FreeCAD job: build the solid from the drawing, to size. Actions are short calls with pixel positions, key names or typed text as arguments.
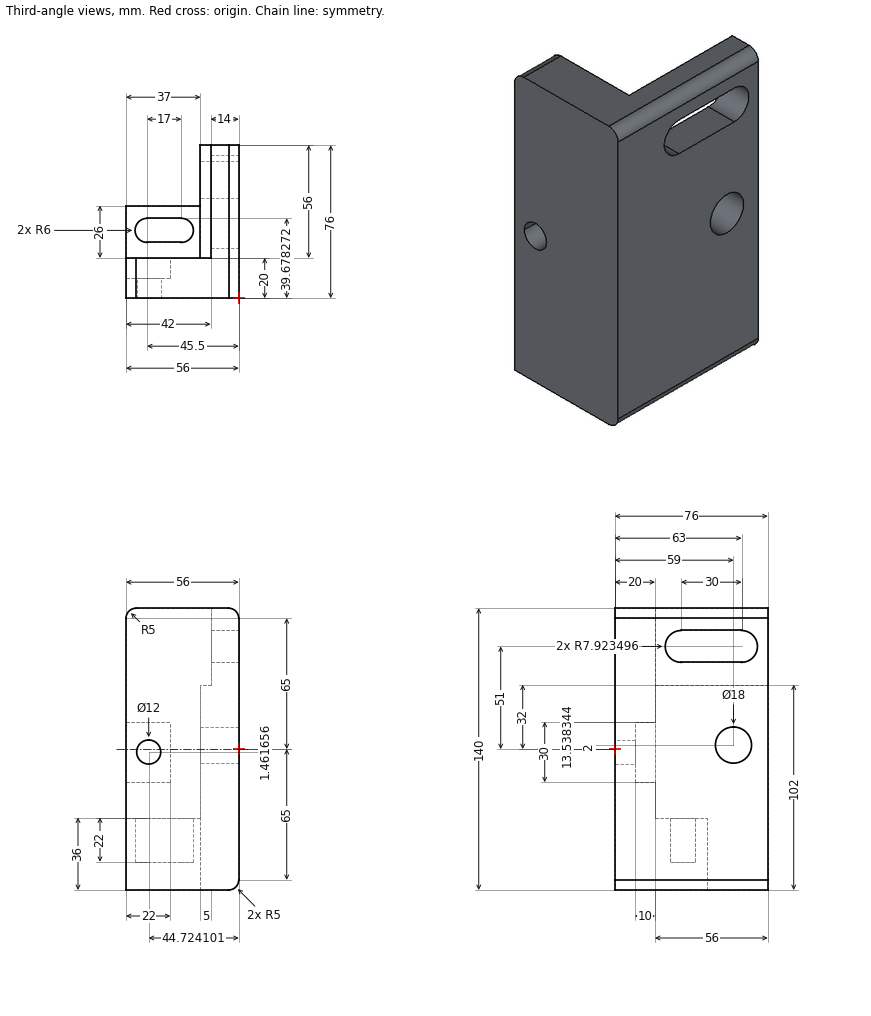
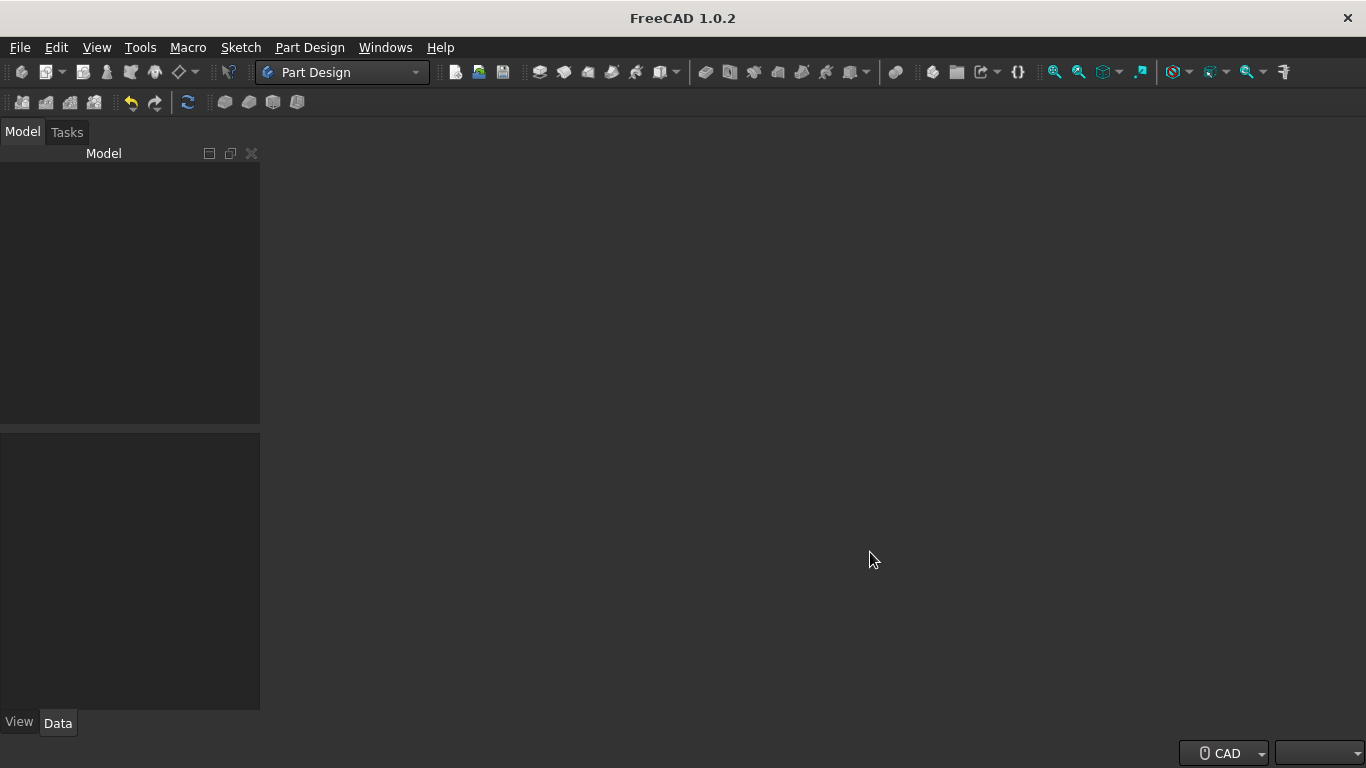
key(ctrl+n)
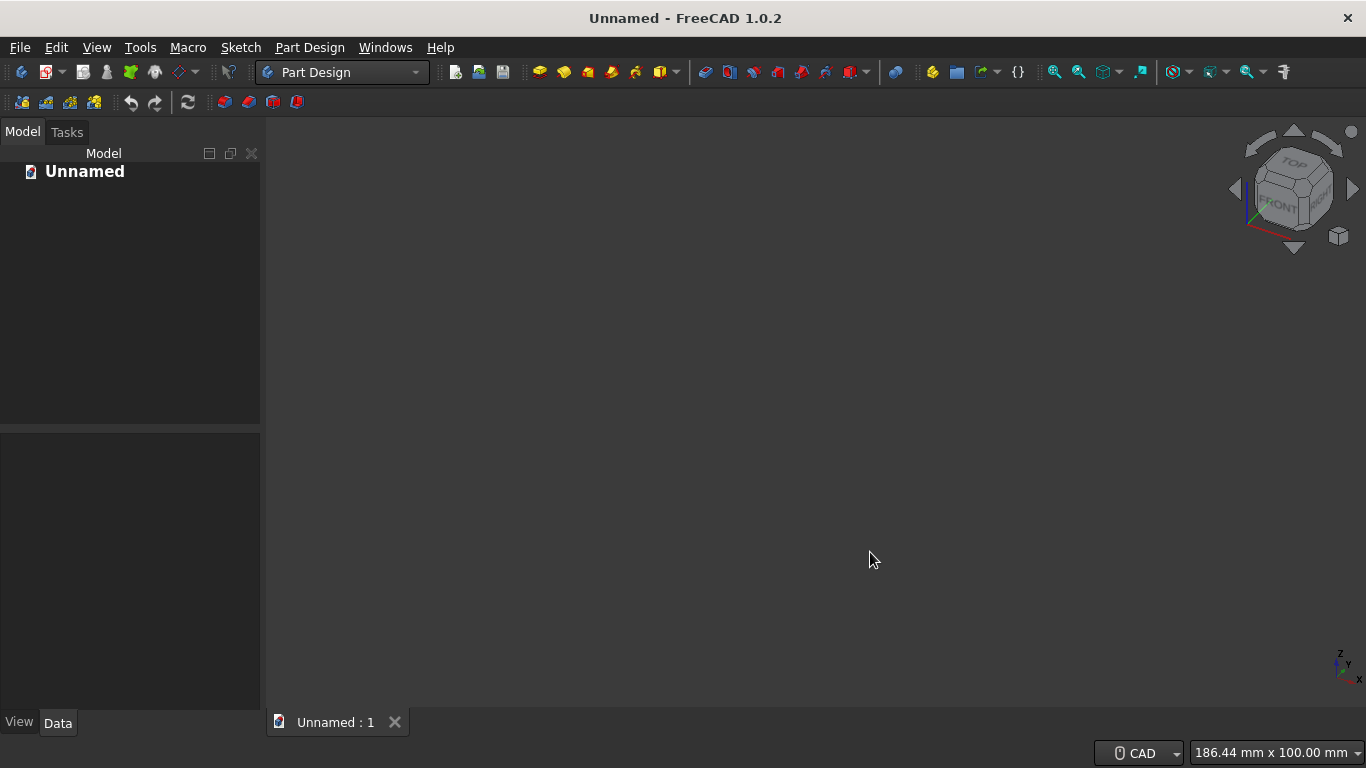
click(46, 72)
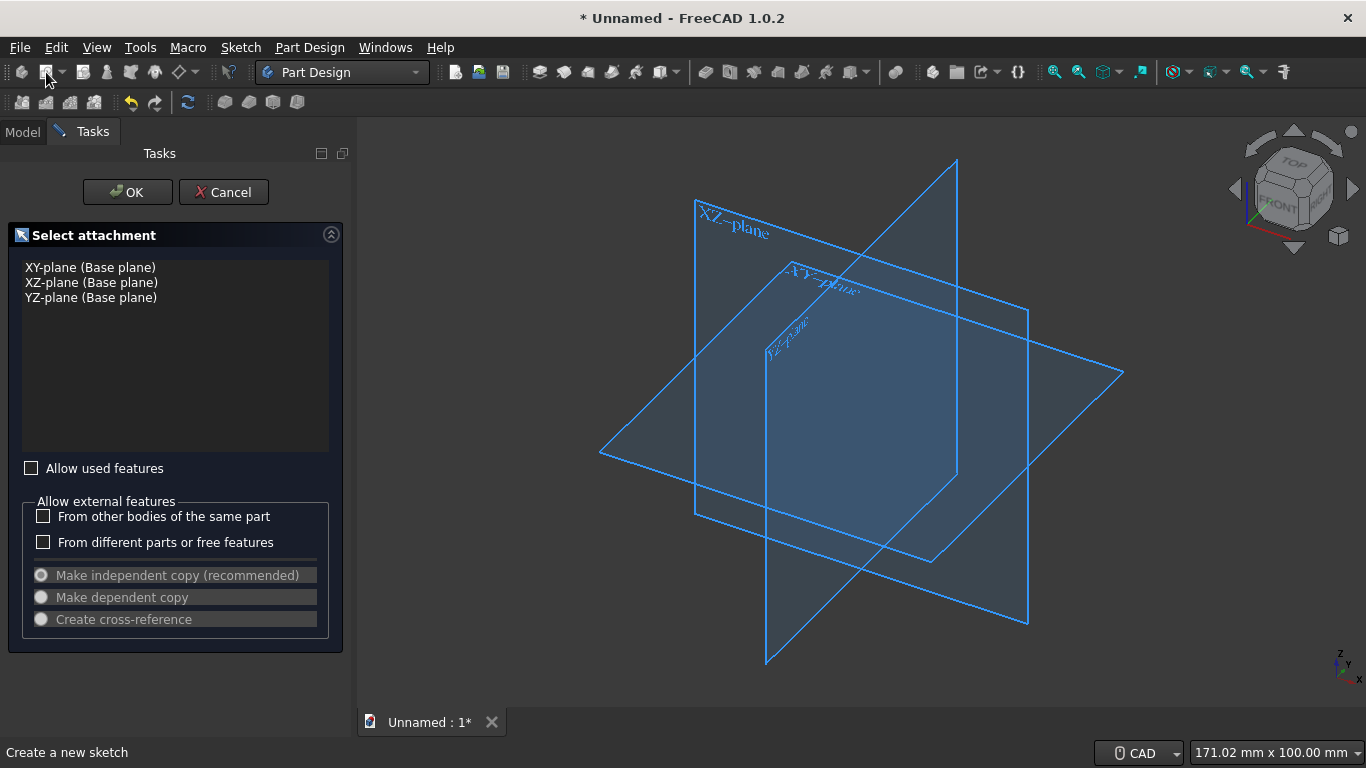
click(82, 268)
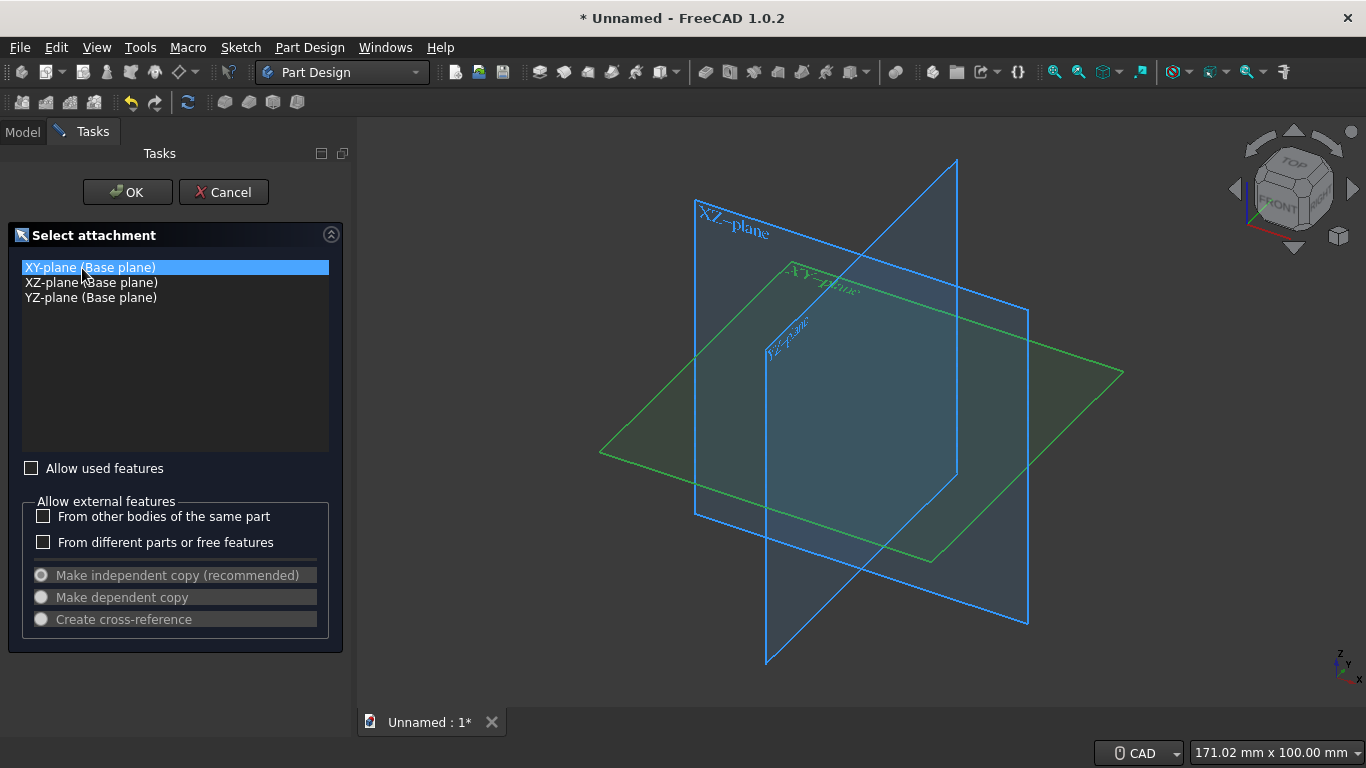
click(128, 192)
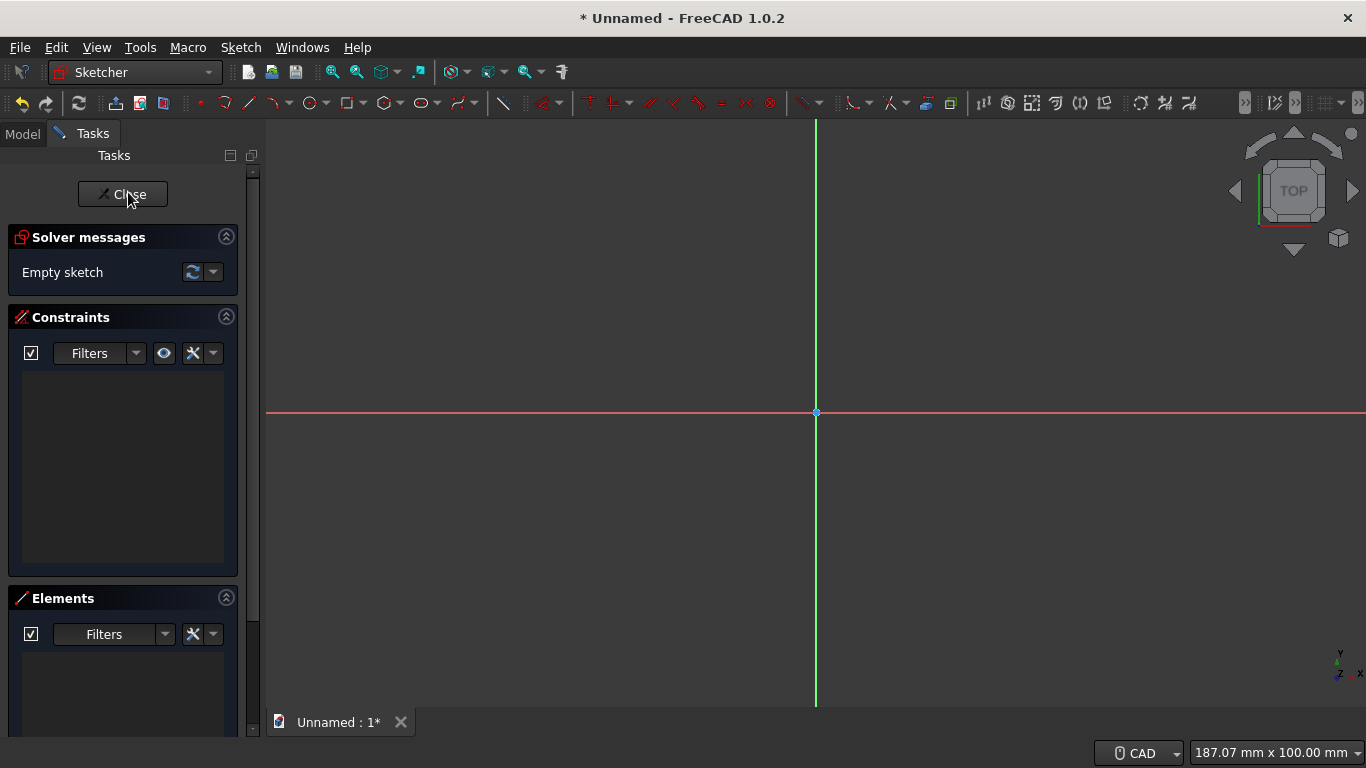
scroll(943, 679, down, 2)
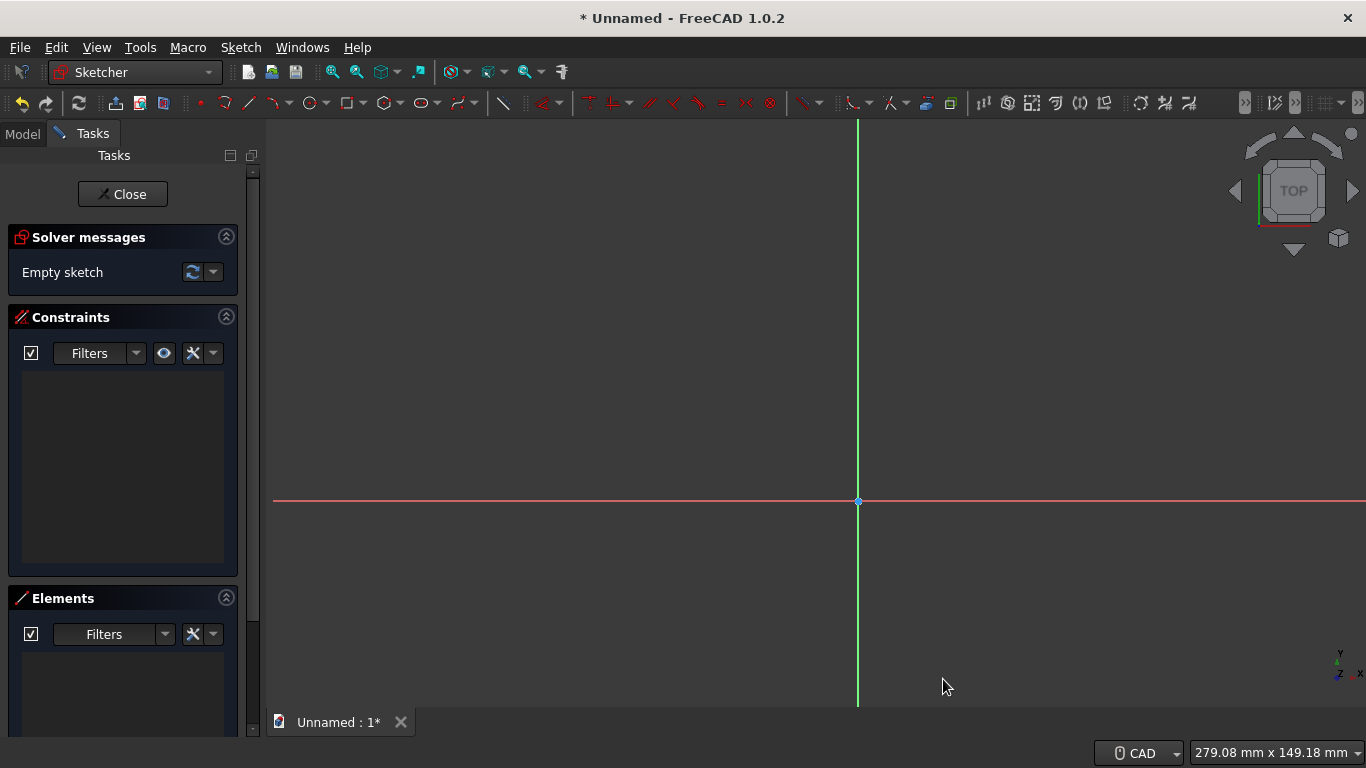
click(226, 104)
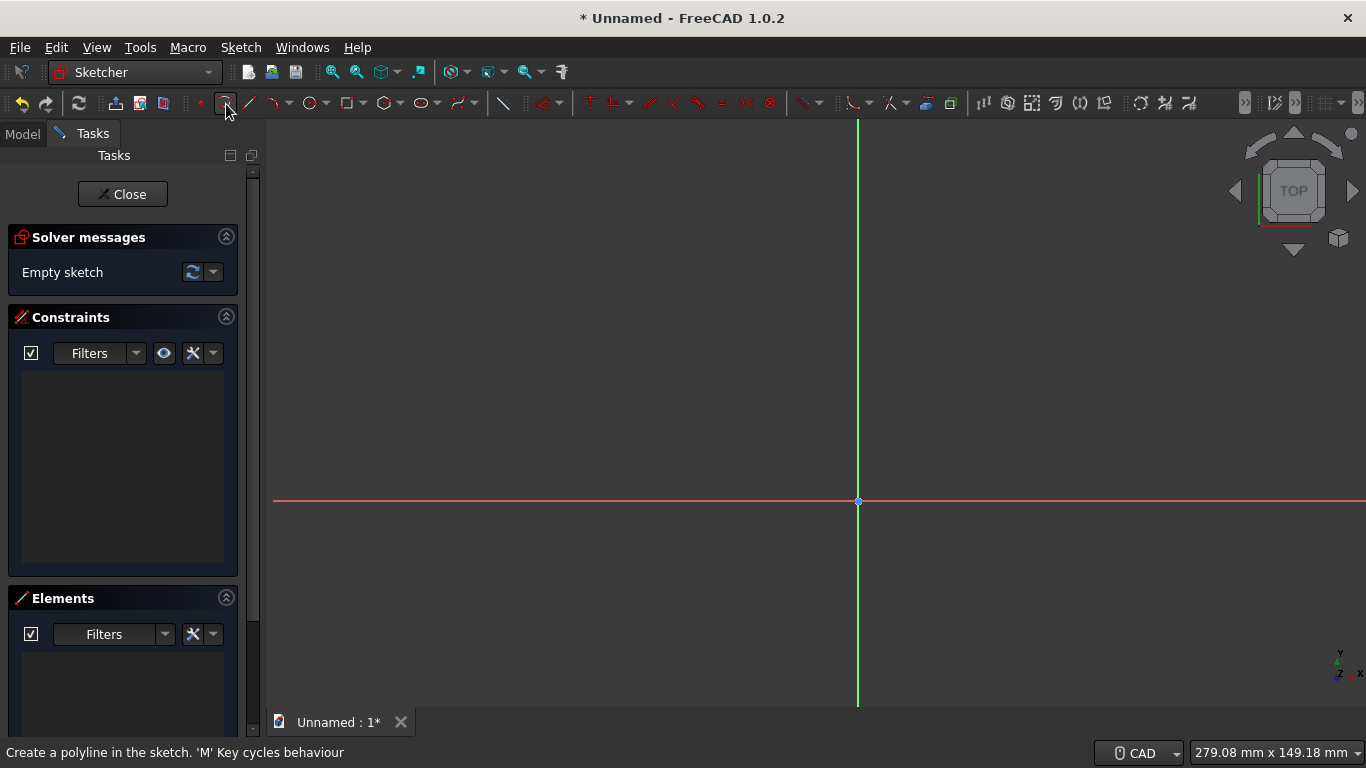
click(858, 501)
click(849, 201)
click(803, 201)
click(803, 422)
click(637, 422)
click(637, 492)
click(858, 501)
key(Escape)
key(Escape)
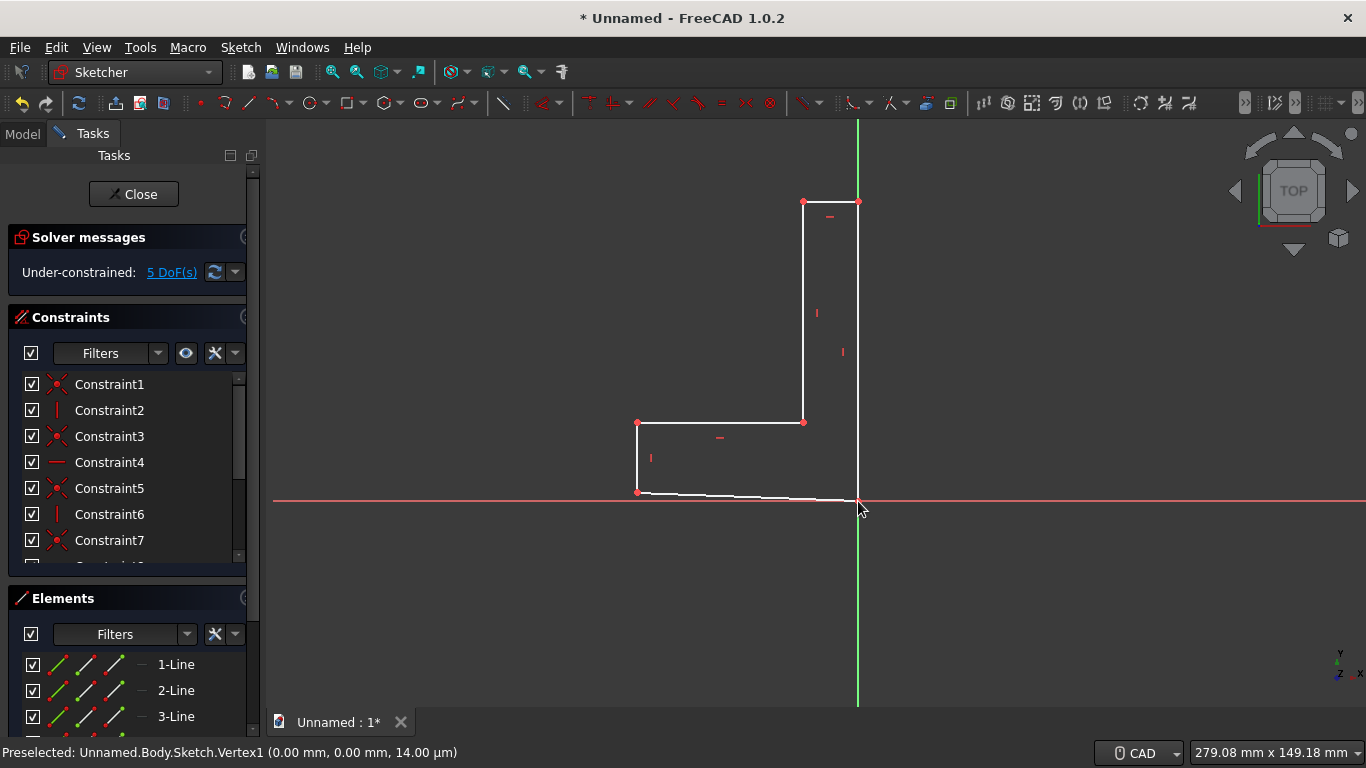
click(792, 499)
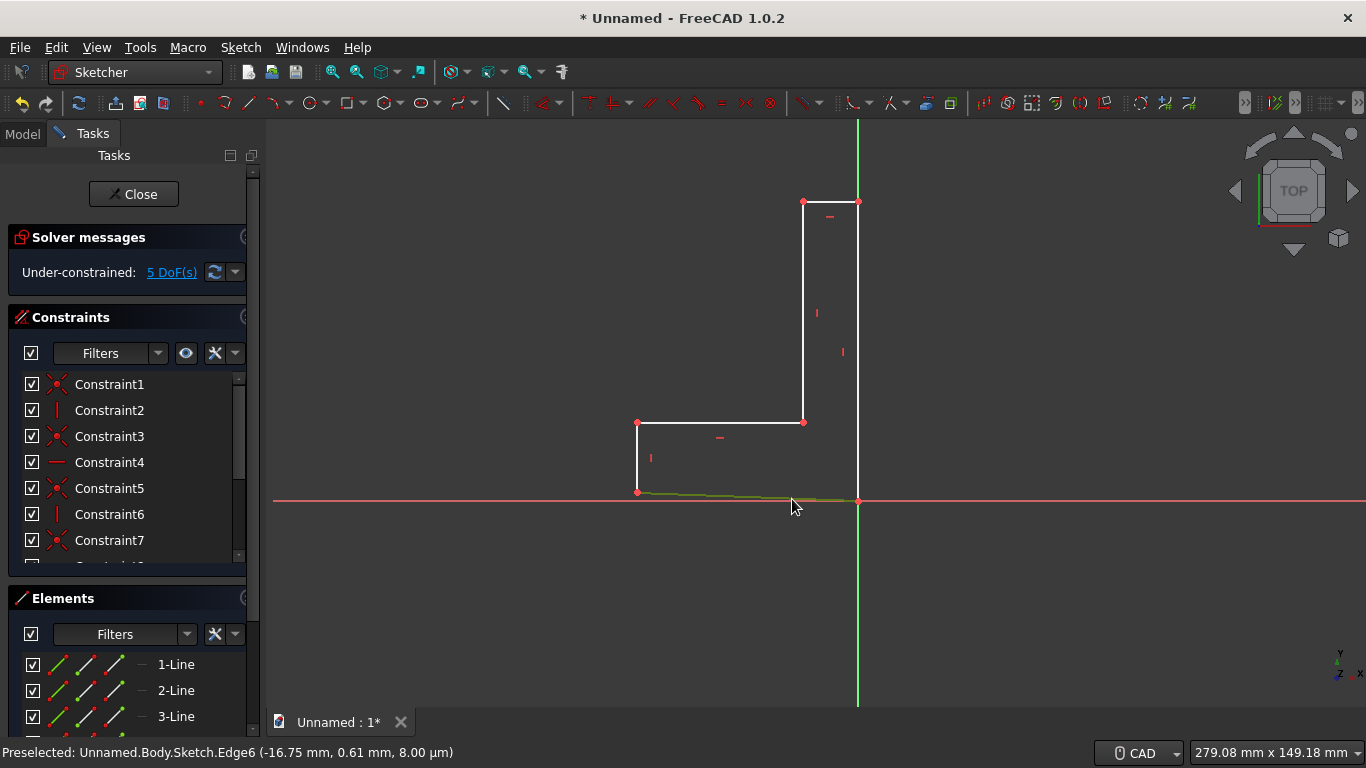
key(h)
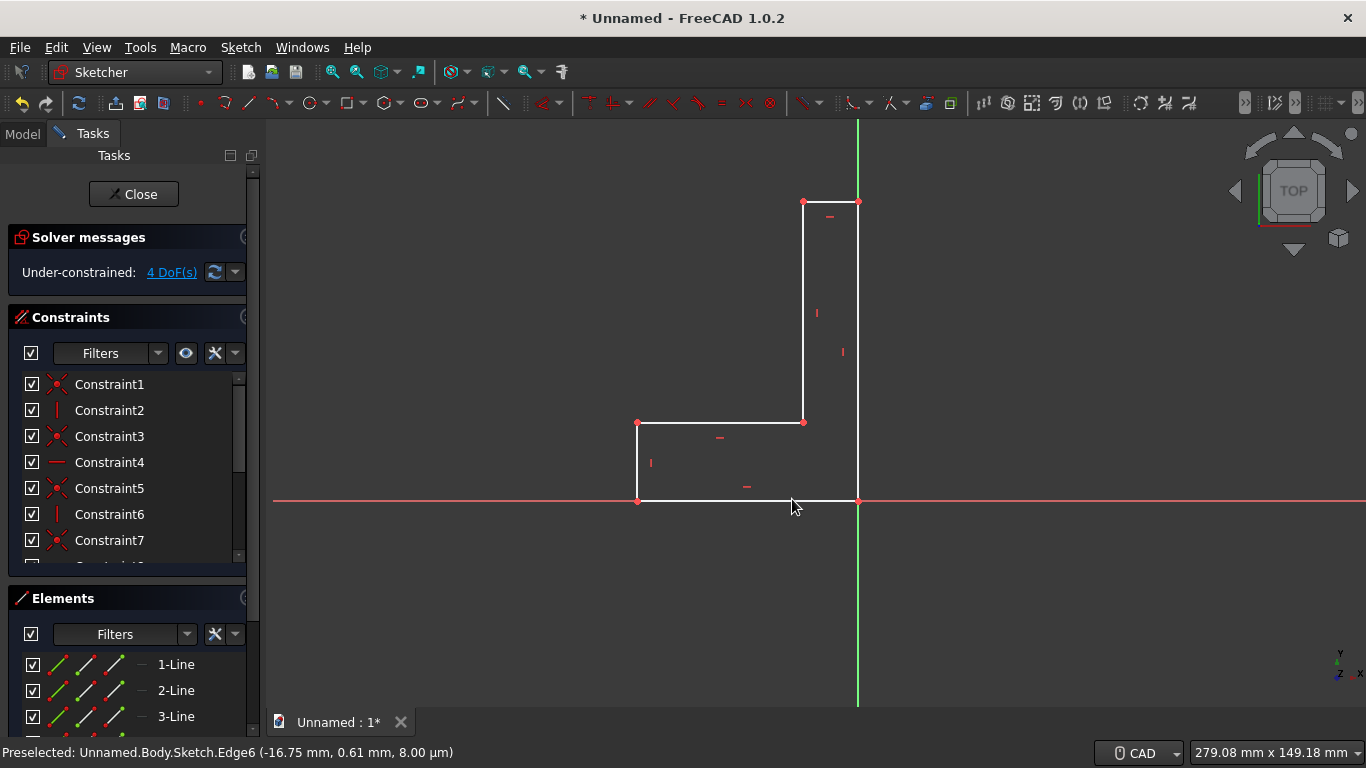
click(542, 104)